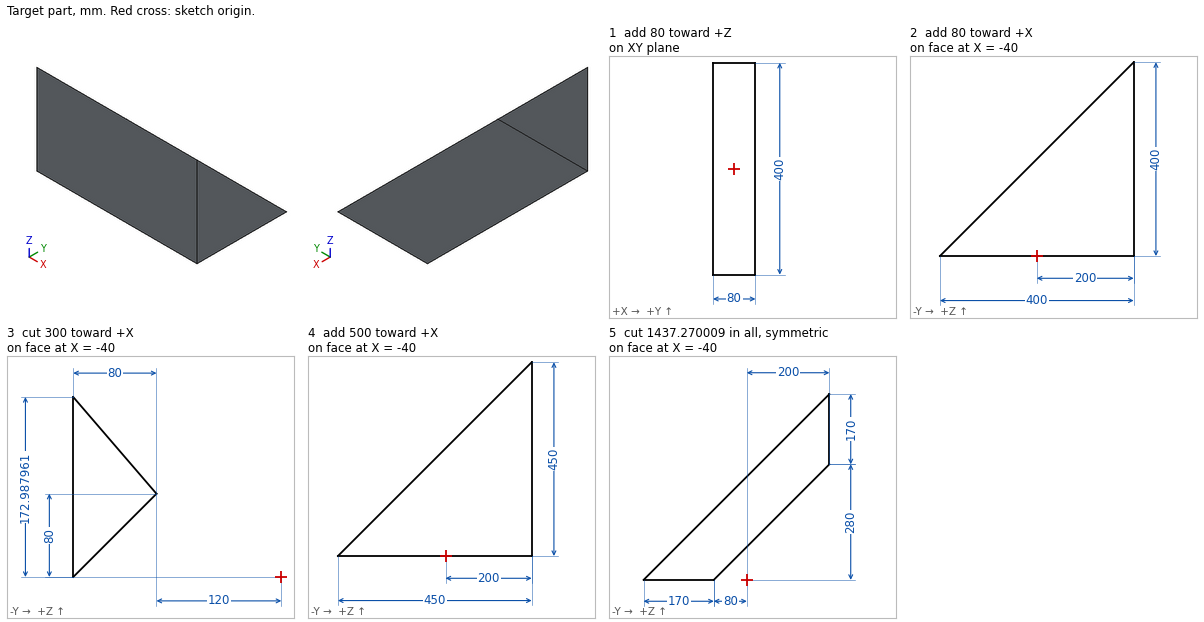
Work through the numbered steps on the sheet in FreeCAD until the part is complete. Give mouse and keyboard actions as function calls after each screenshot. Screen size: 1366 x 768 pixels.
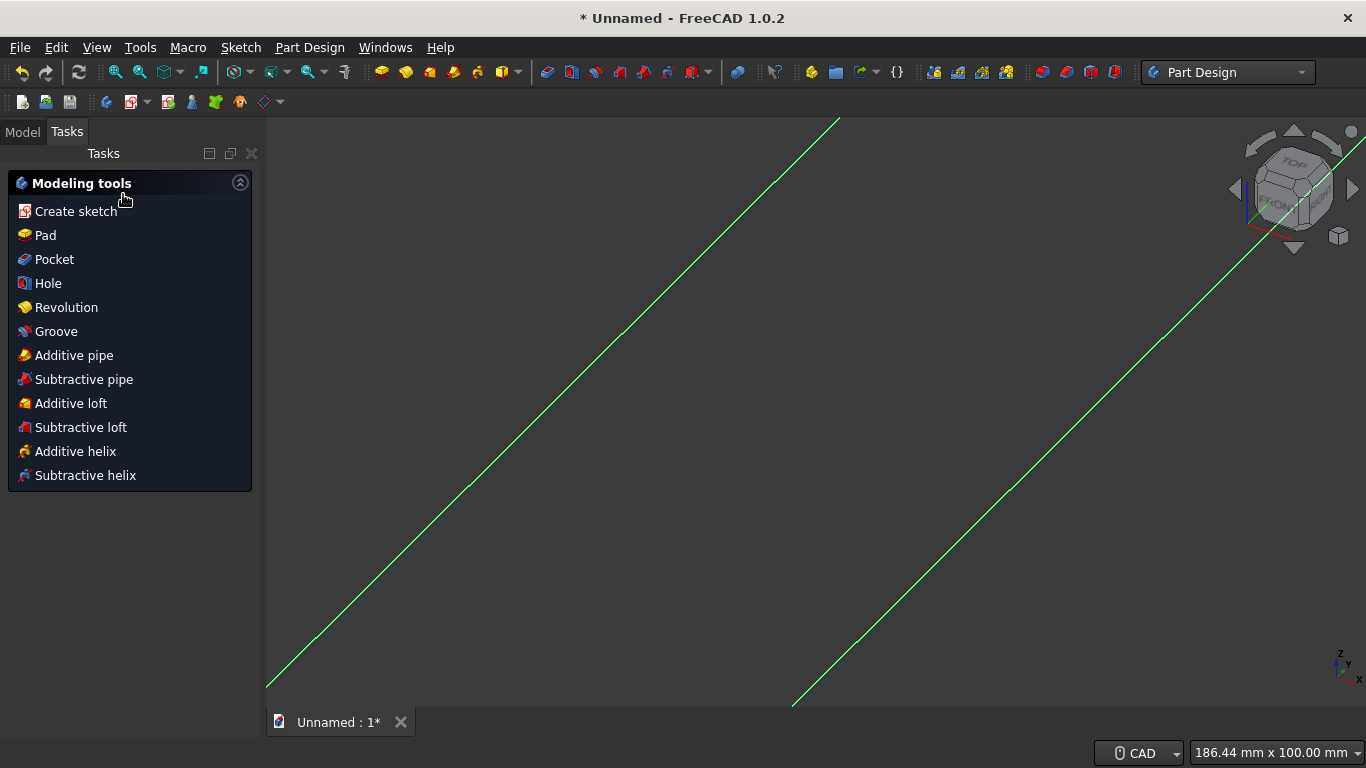
click(382, 72)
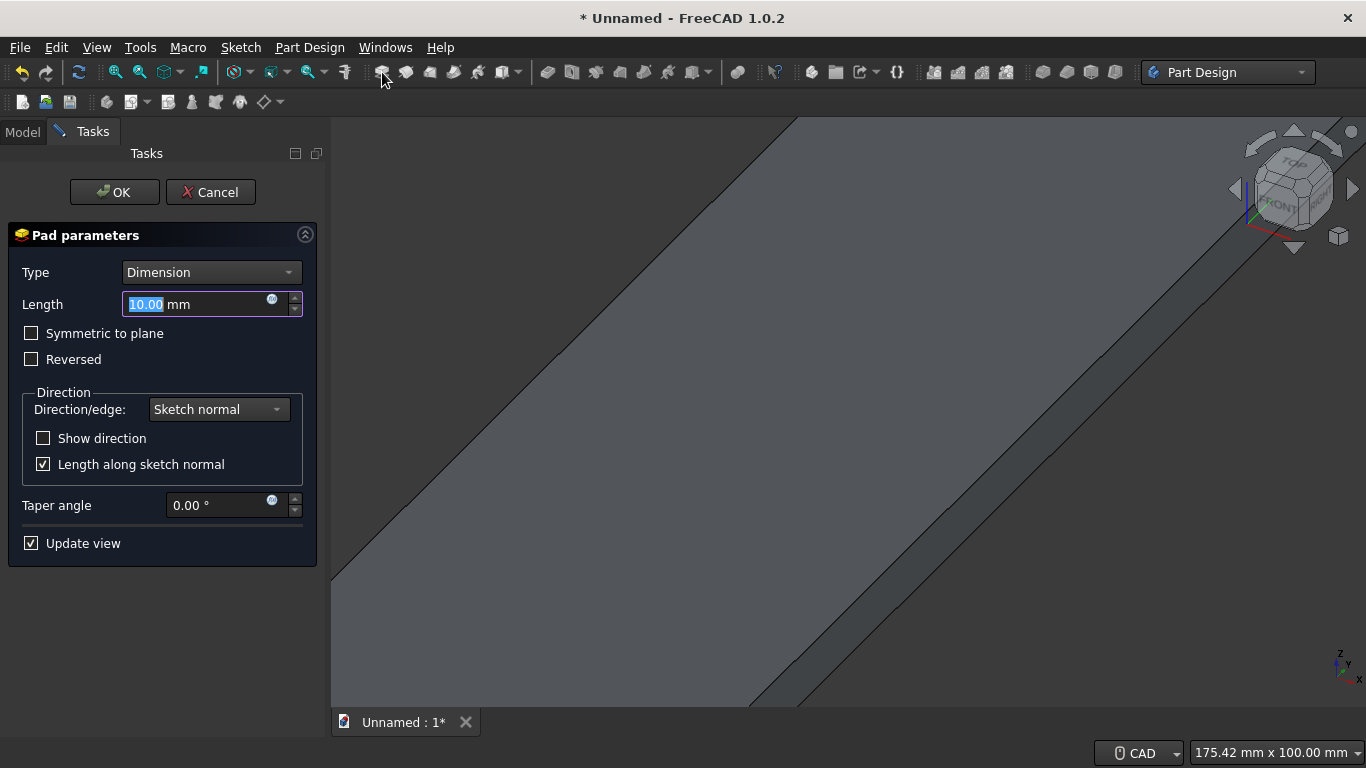
text(80)
key(Tab)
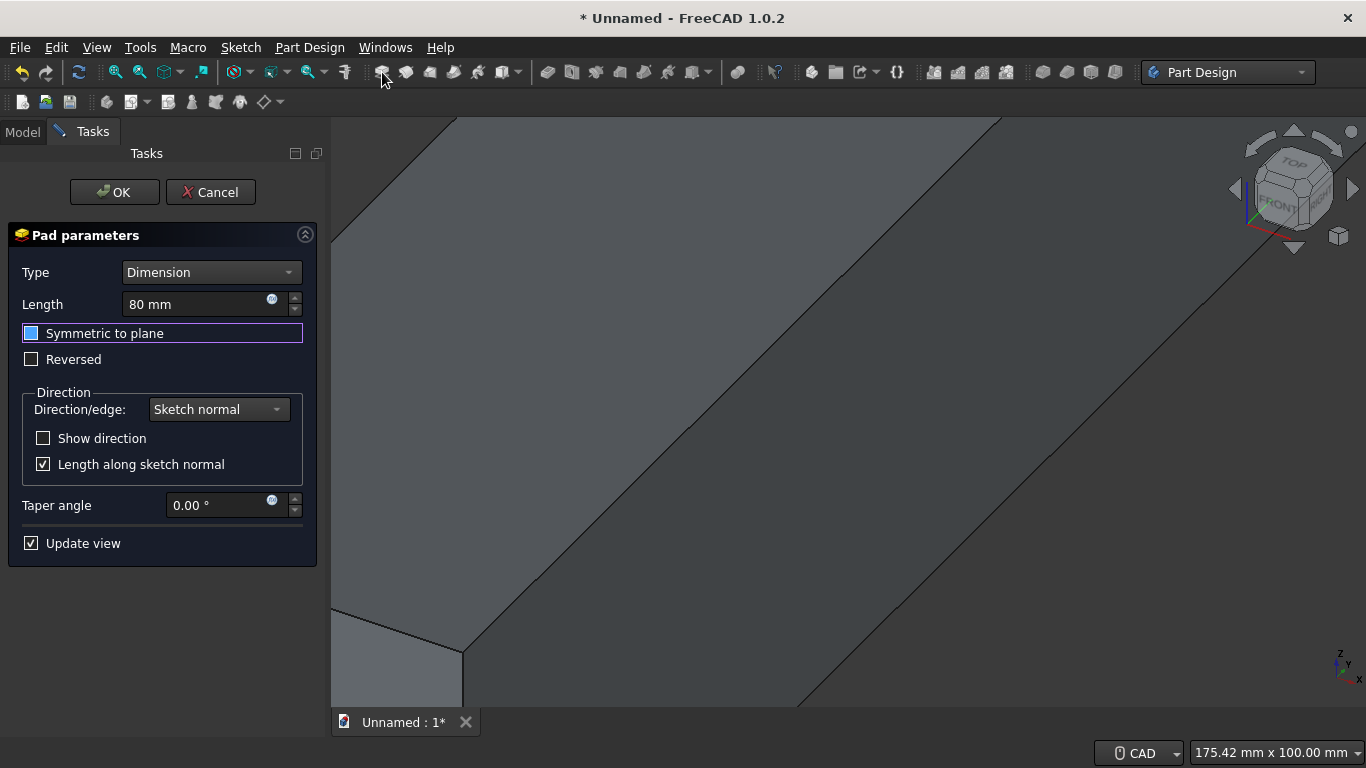
click(115, 192)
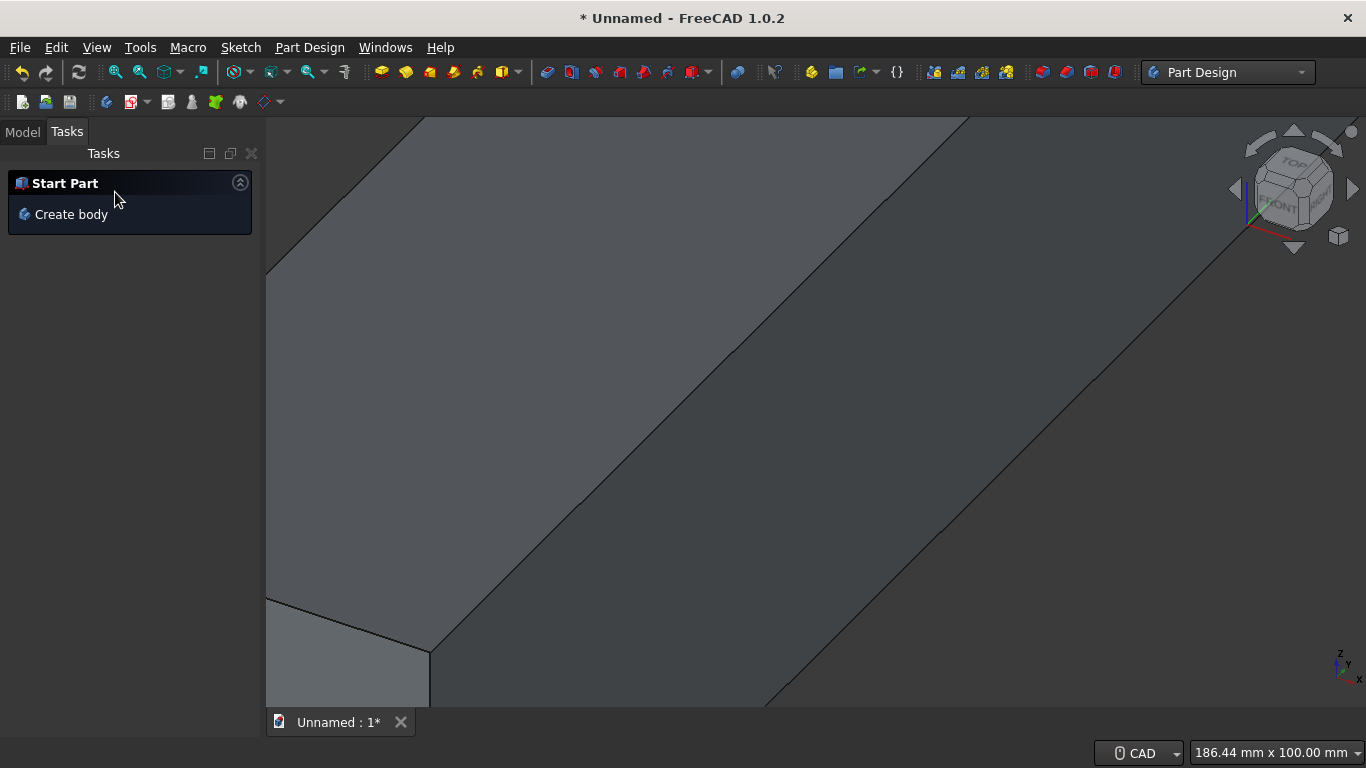
click(116, 72)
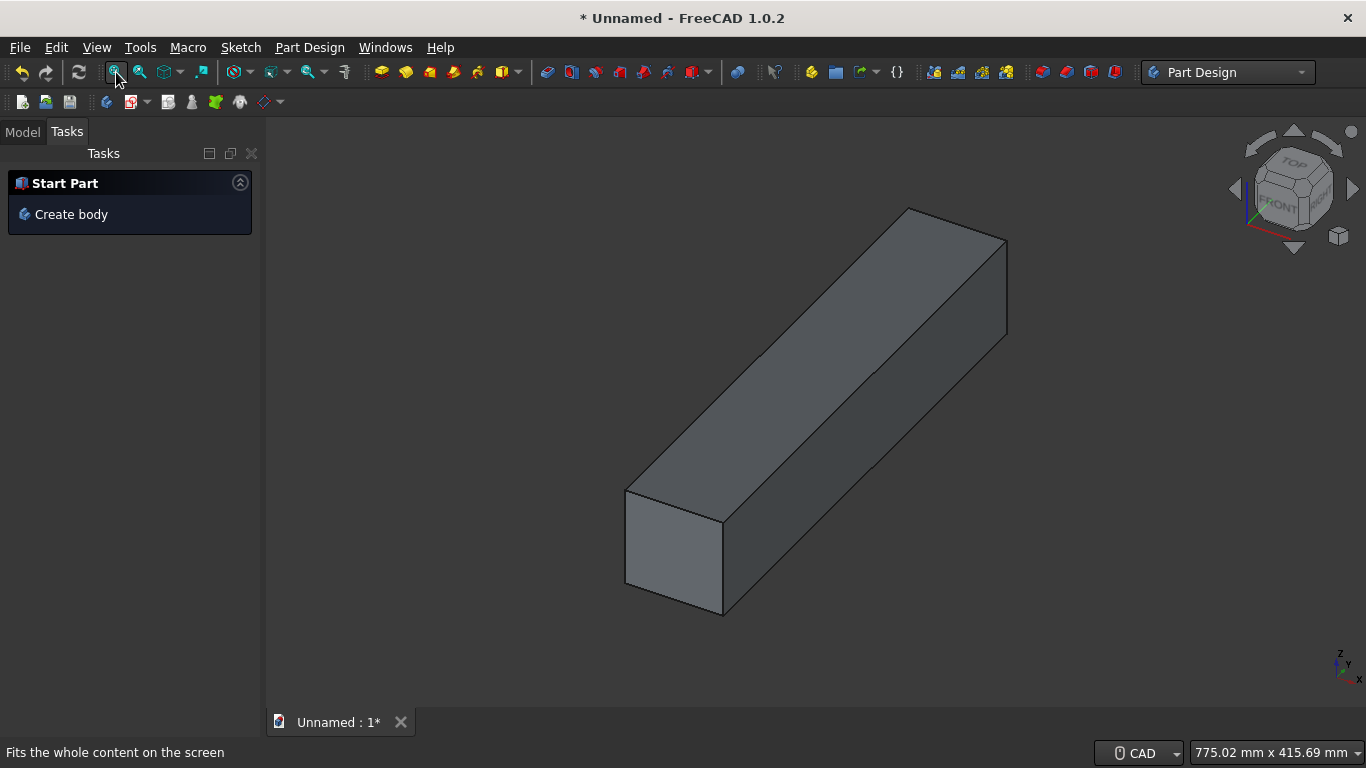
key(6)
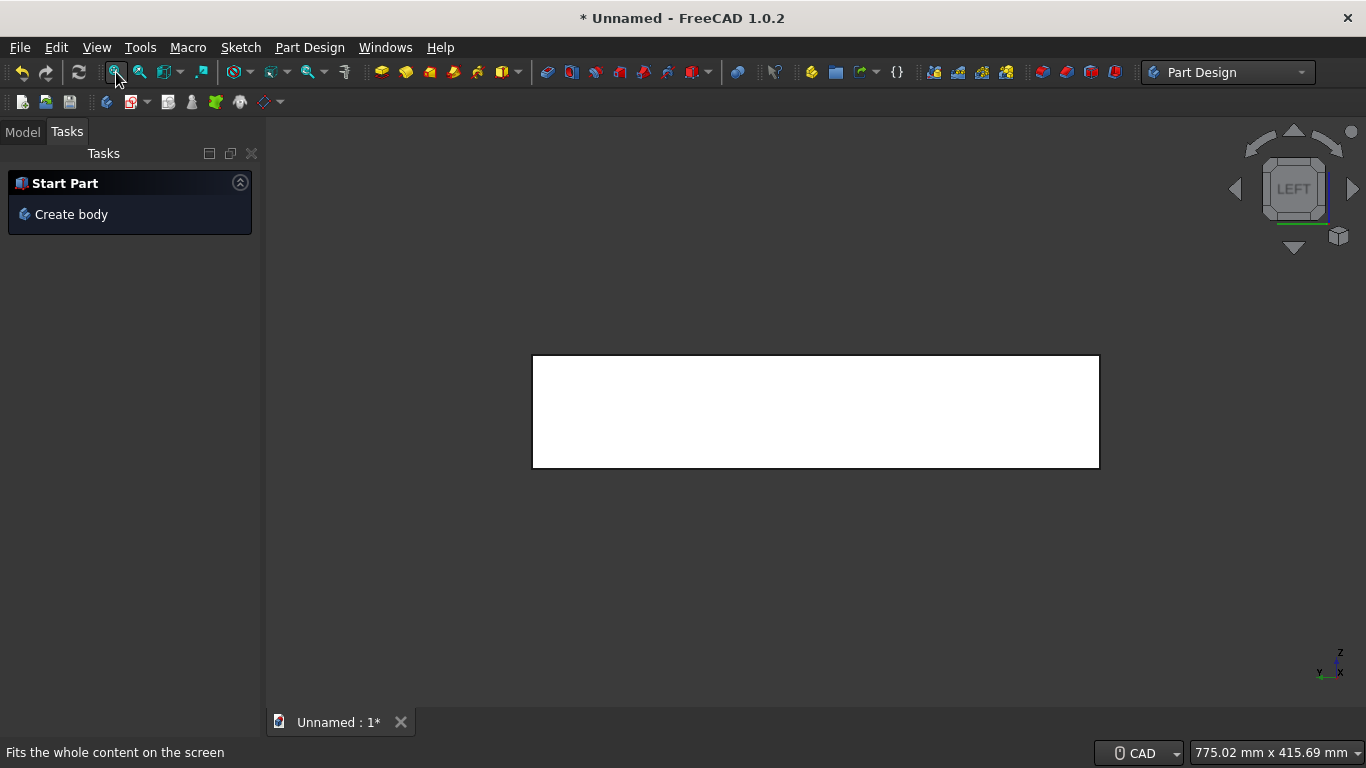
click(654, 411)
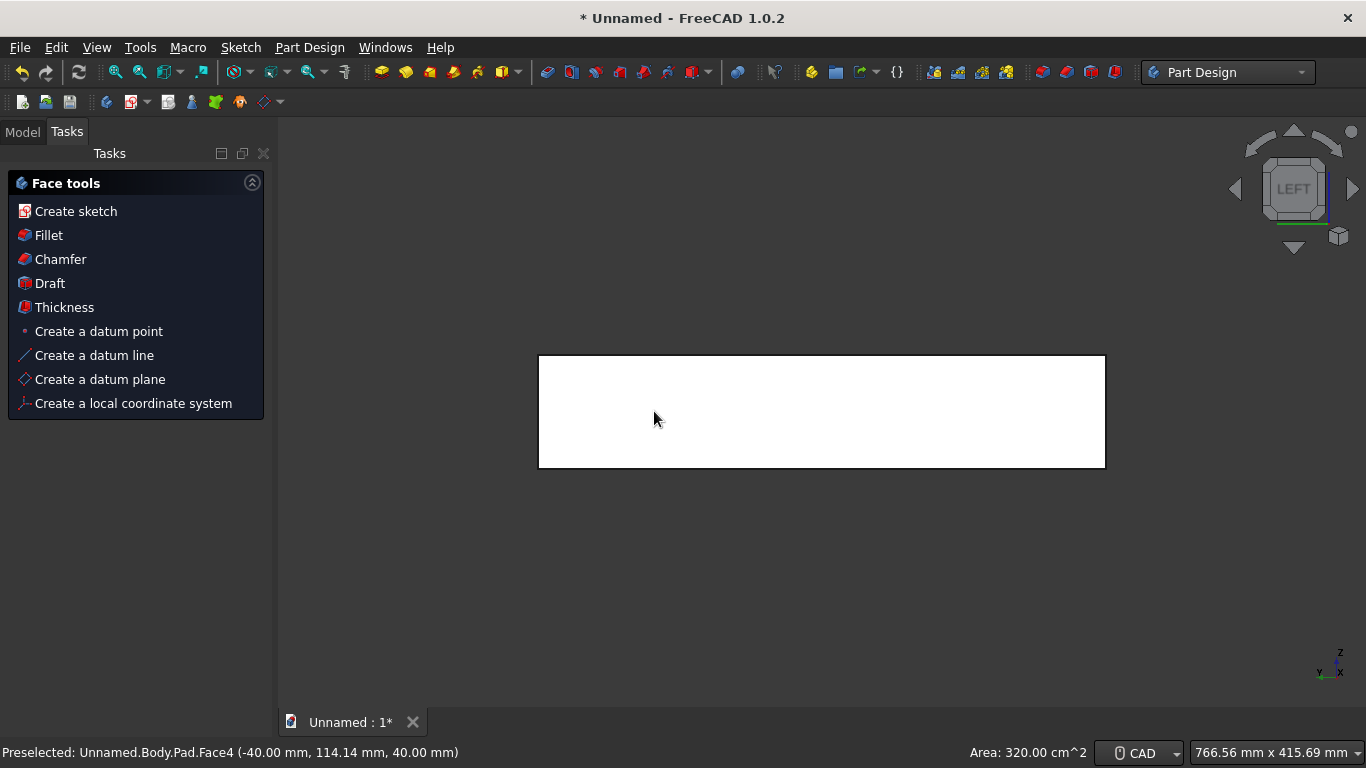
click(132, 102)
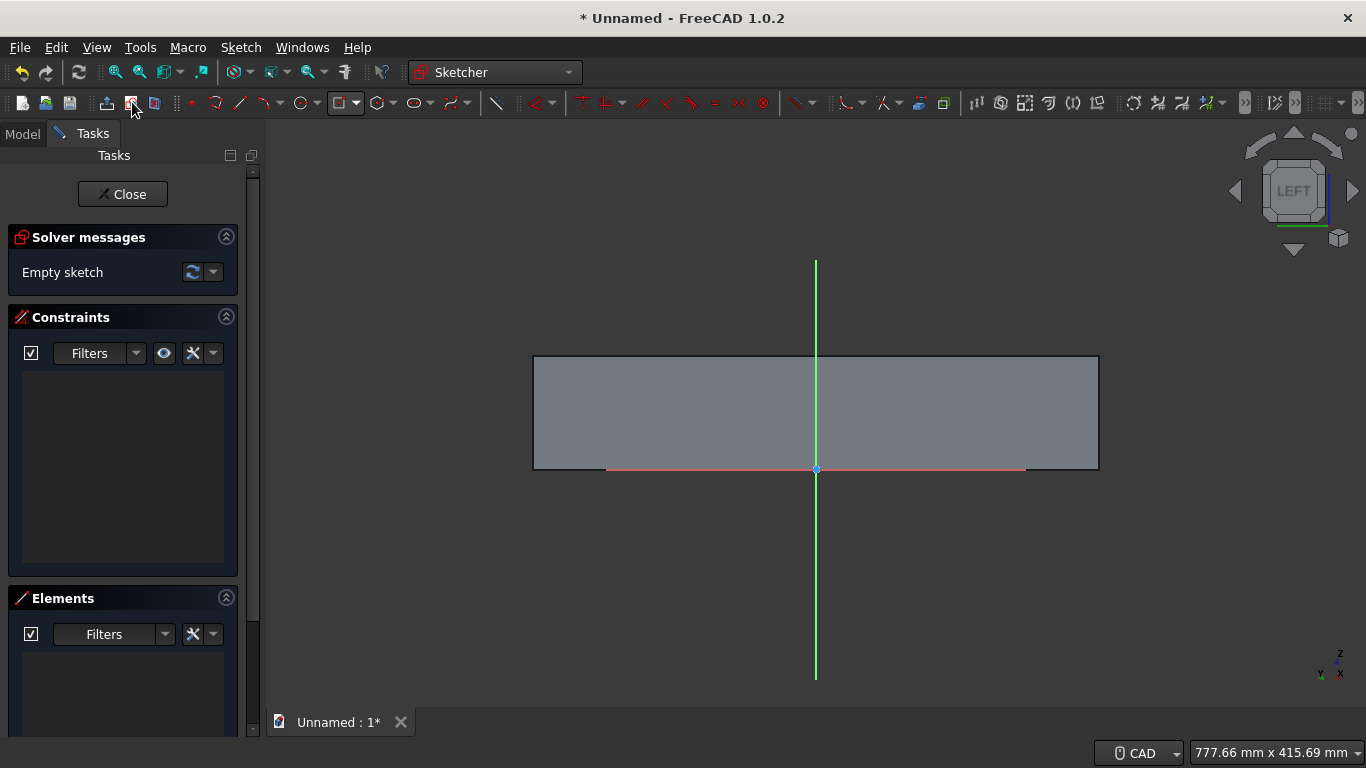
scroll(664, 679, down, 3)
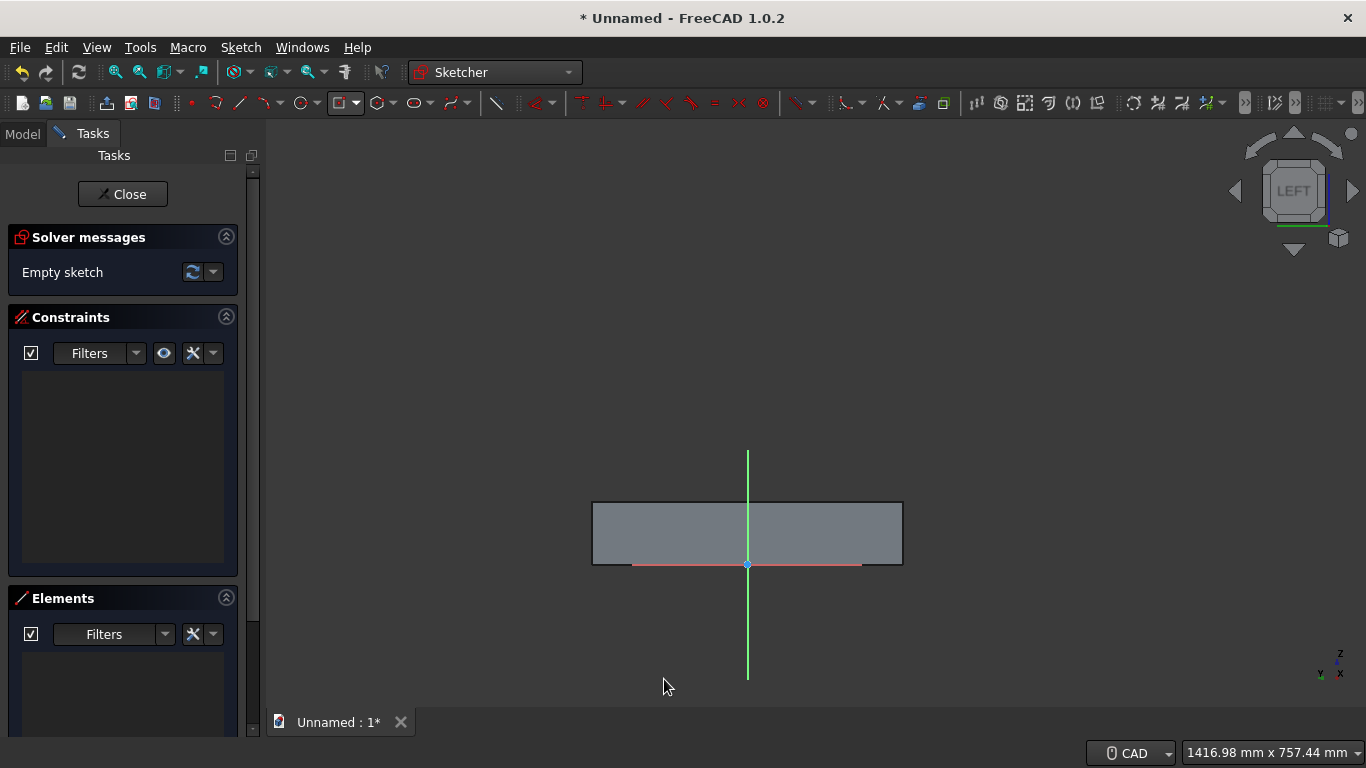
click(216, 104)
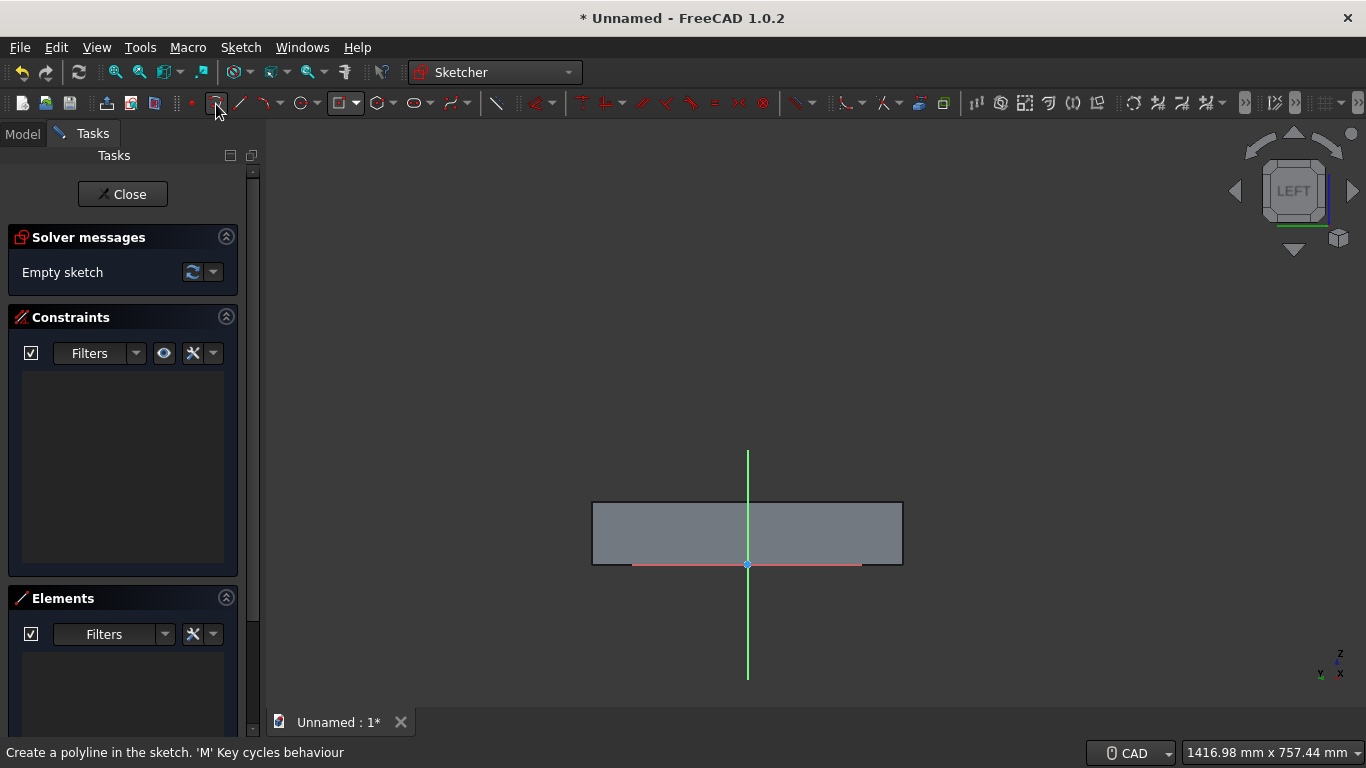
click(903, 564)
click(903, 254)
click(592, 555)
click(903, 565)
key(Escape)
key(Escape)